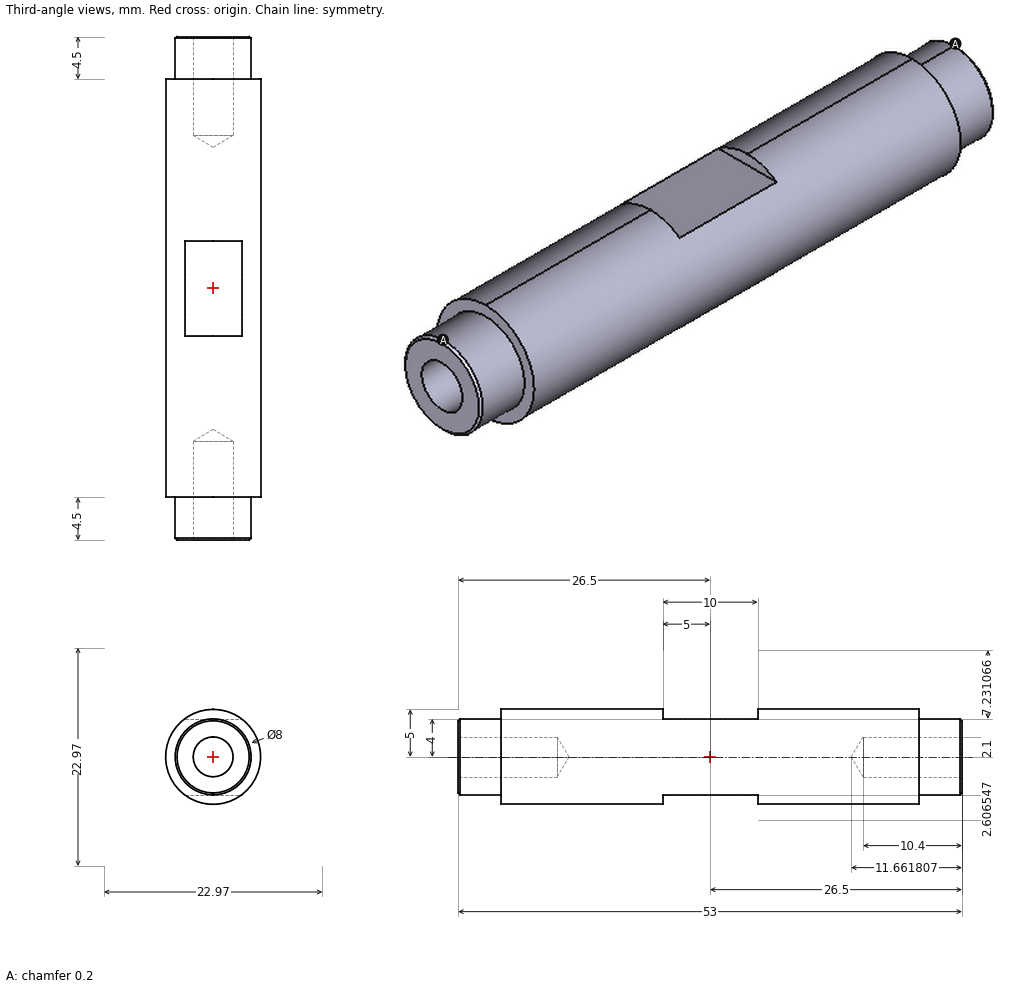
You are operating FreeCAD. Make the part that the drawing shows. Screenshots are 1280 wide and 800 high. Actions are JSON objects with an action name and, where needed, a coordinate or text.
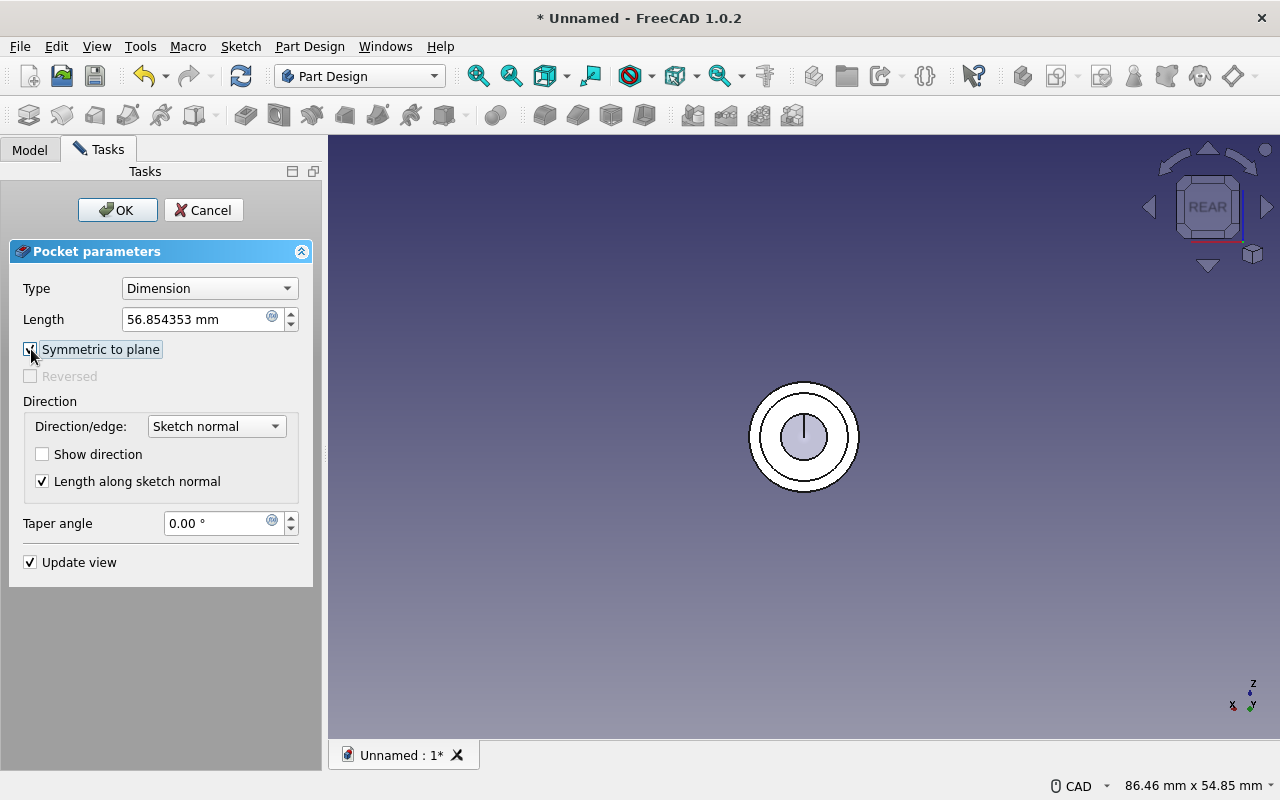
{"action": "left_click", "coordinate": [118, 210]}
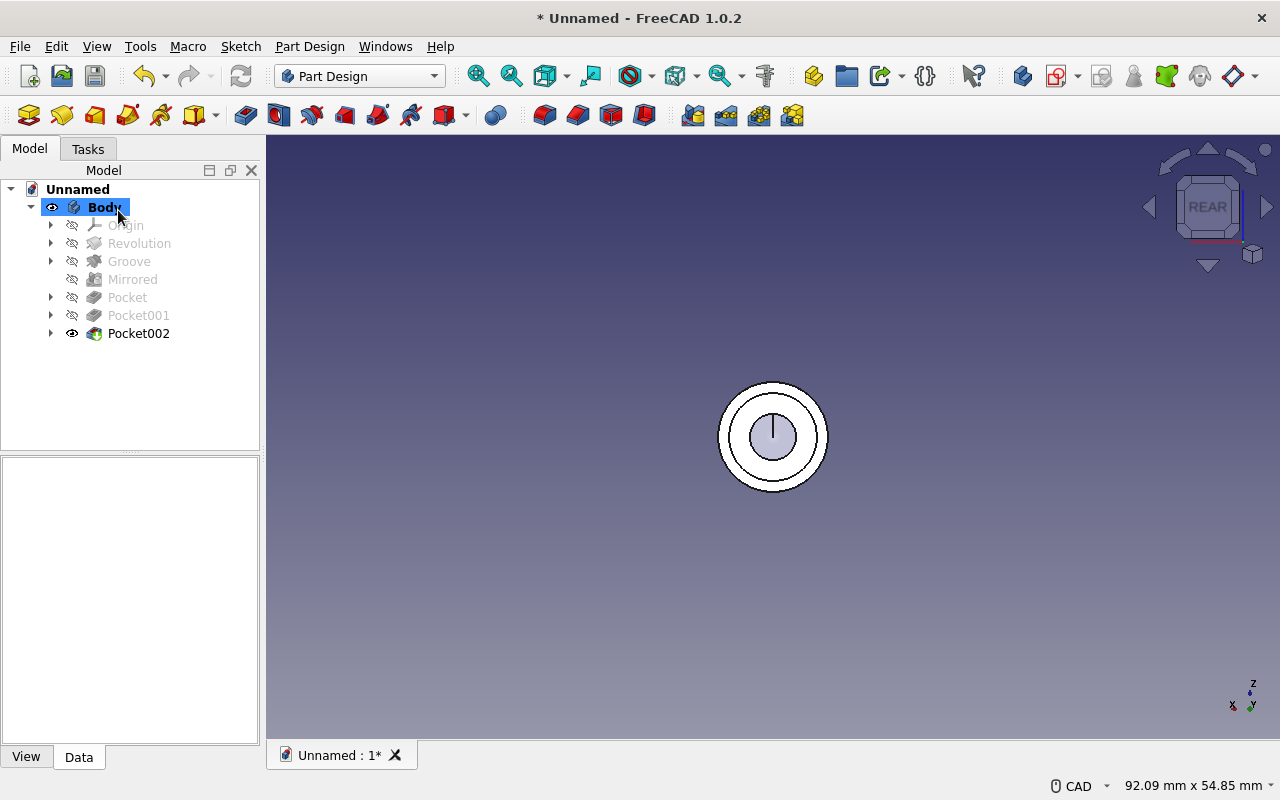
{"action": "left_click", "coordinate": [479, 76]}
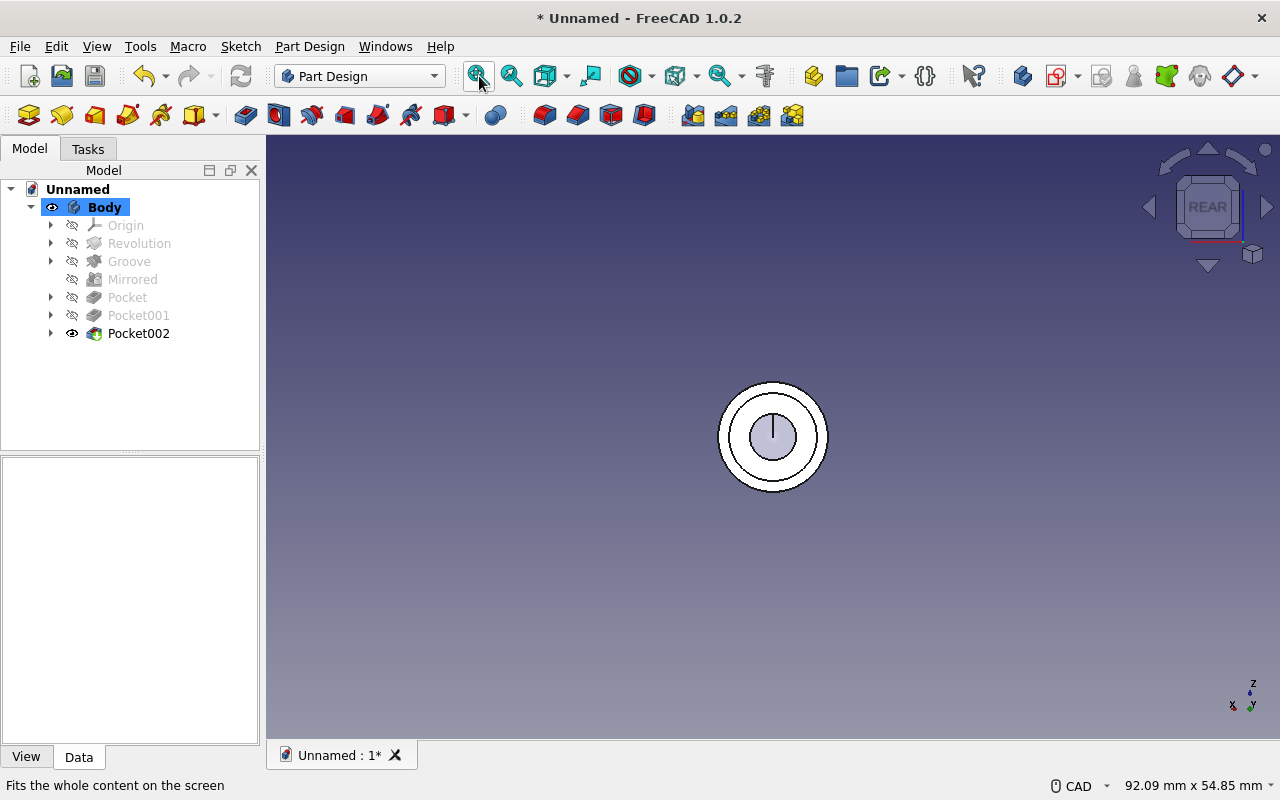
{"action": "left_click", "coordinate": [773, 480]}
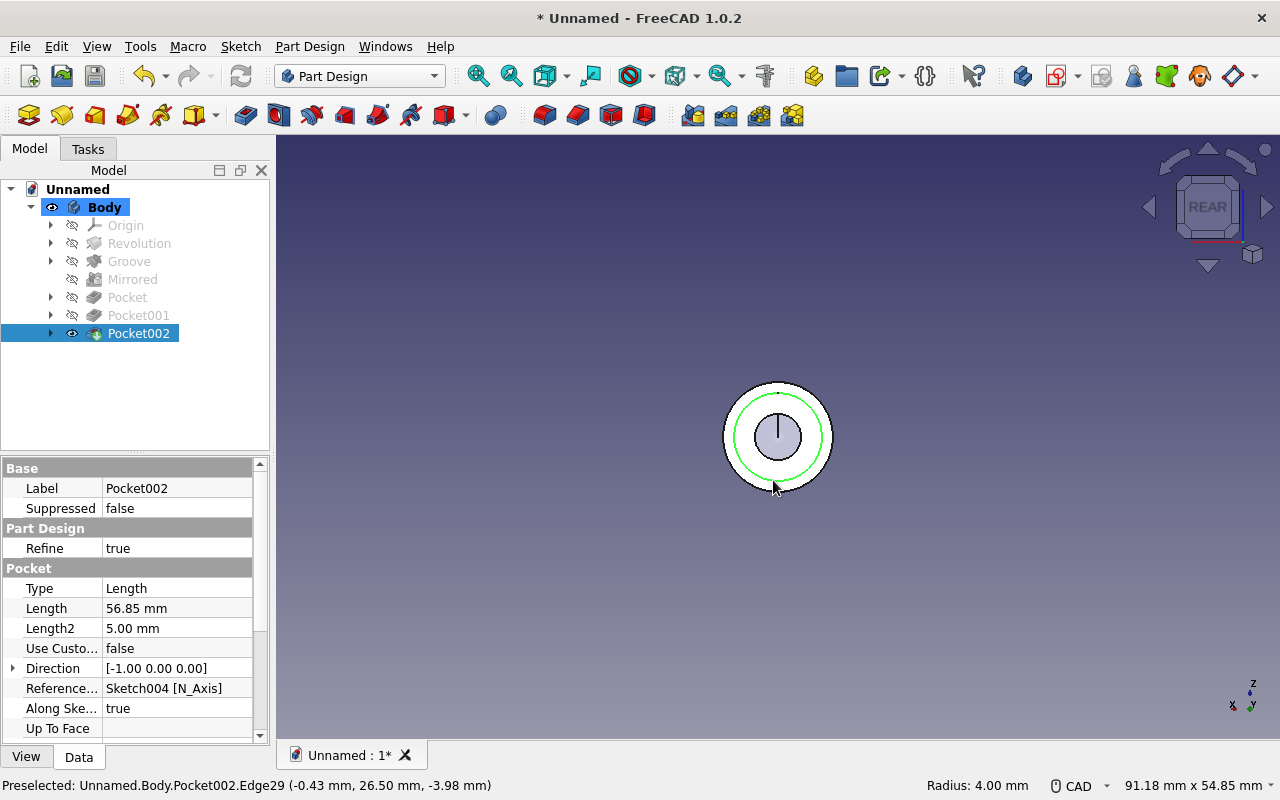
{"action": "key", "text": "0"}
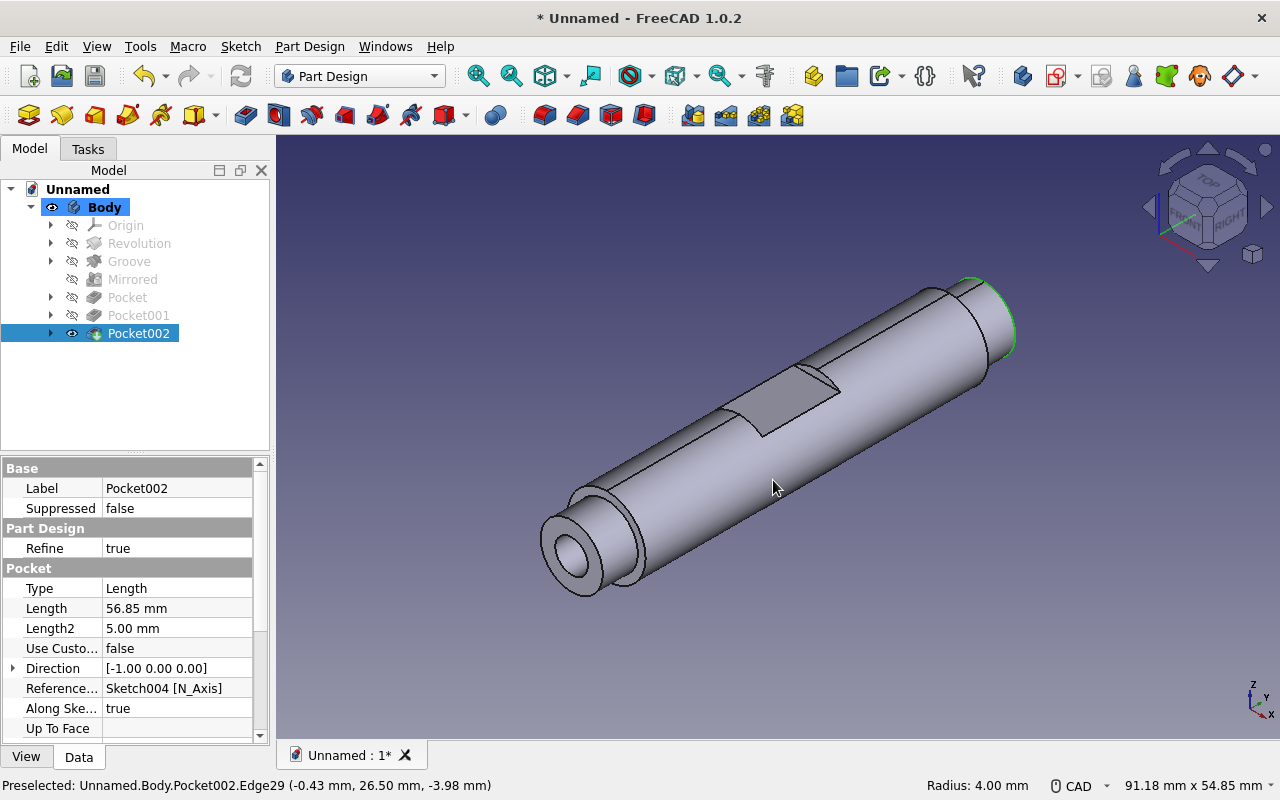
{"action": "left_click", "coordinate": [572, 519], "text": "ctrl"}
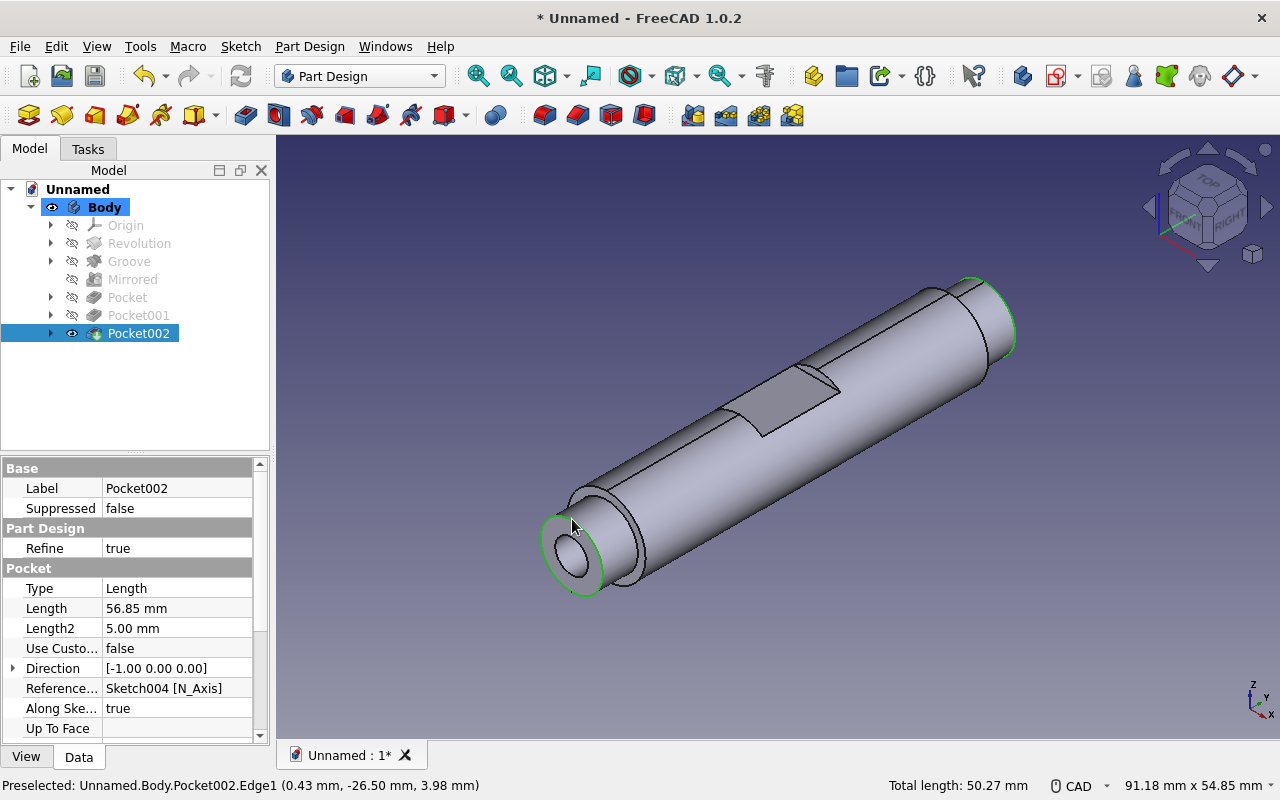
{"action": "left_click", "coordinate": [578, 116]}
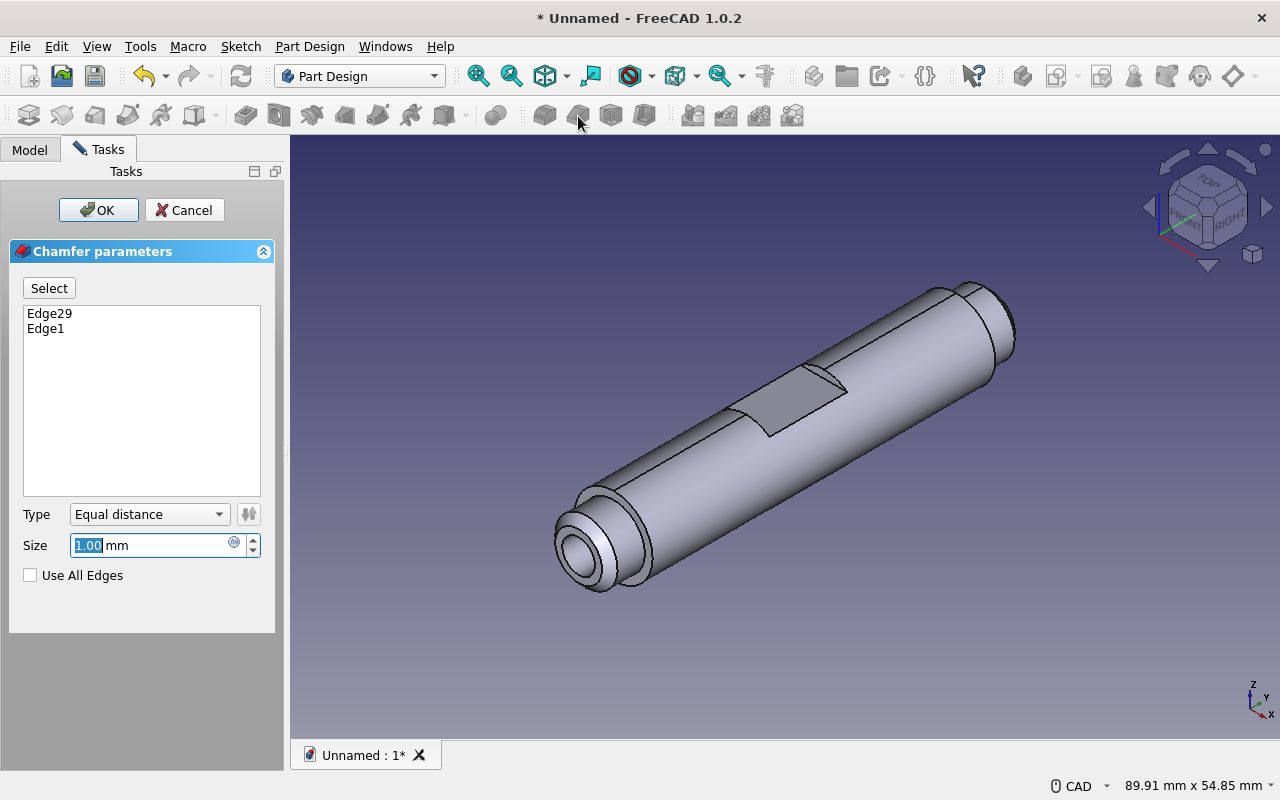
{"action": "type", "text": "0.2"}
{"action": "key", "text": "Tab"}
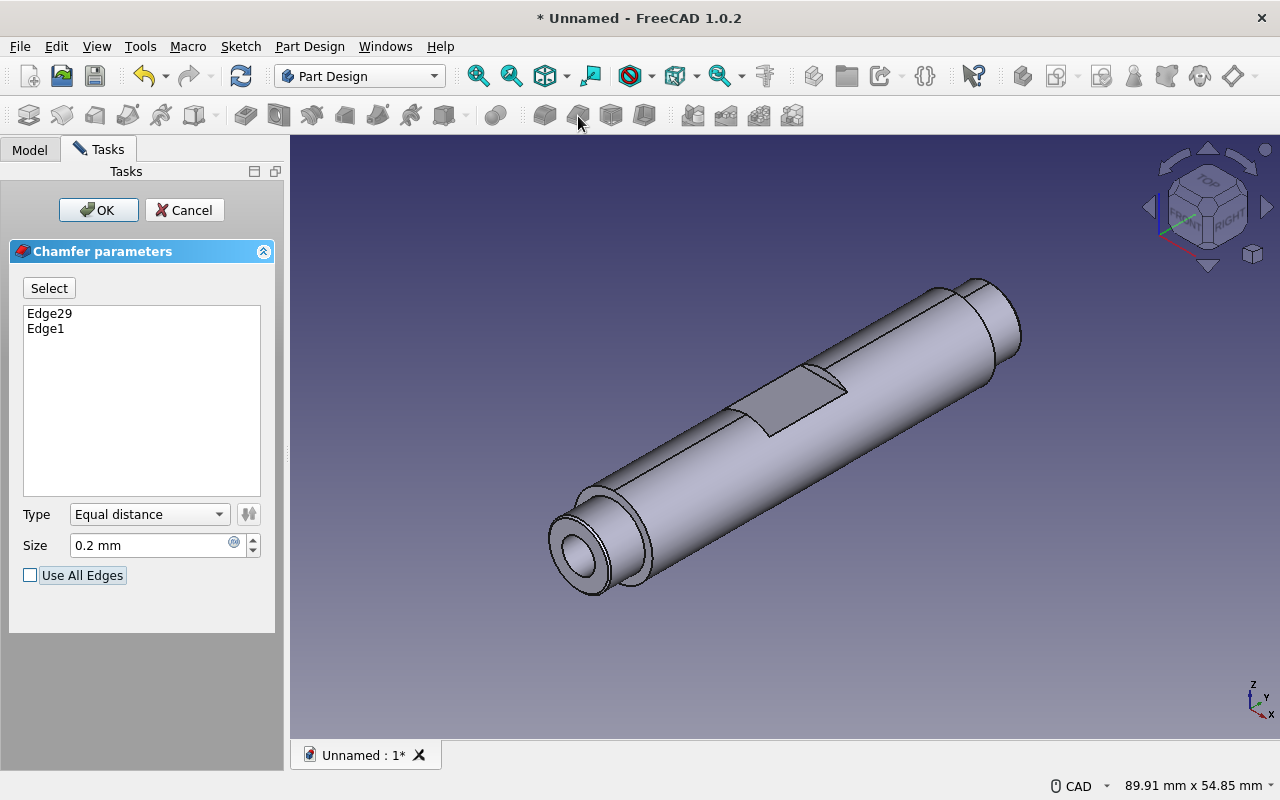
{"action": "left_click", "coordinate": [99, 210]}